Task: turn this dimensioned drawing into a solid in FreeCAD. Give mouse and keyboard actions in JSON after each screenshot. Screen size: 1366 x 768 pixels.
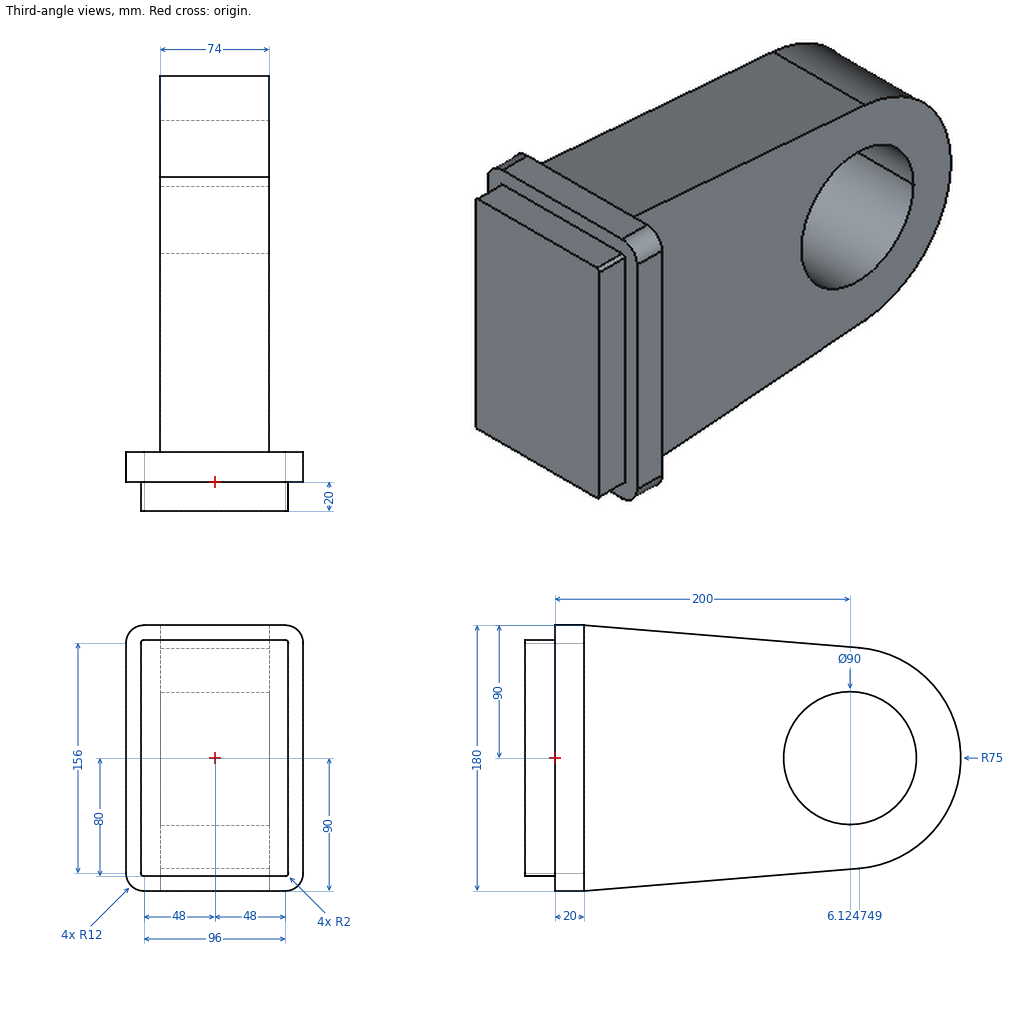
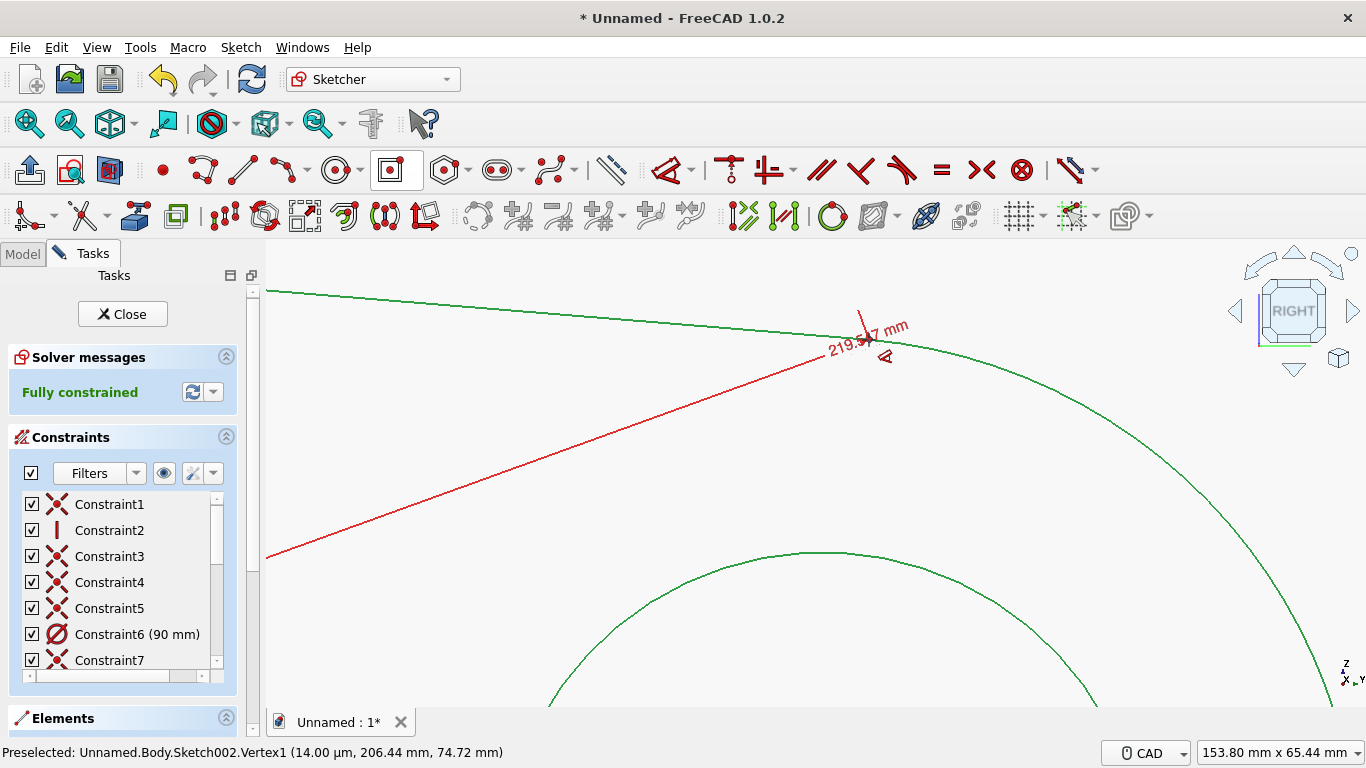
{"action": "scroll", "coordinate": [869, 342], "scroll_direction": "down", "scroll_amount": 7}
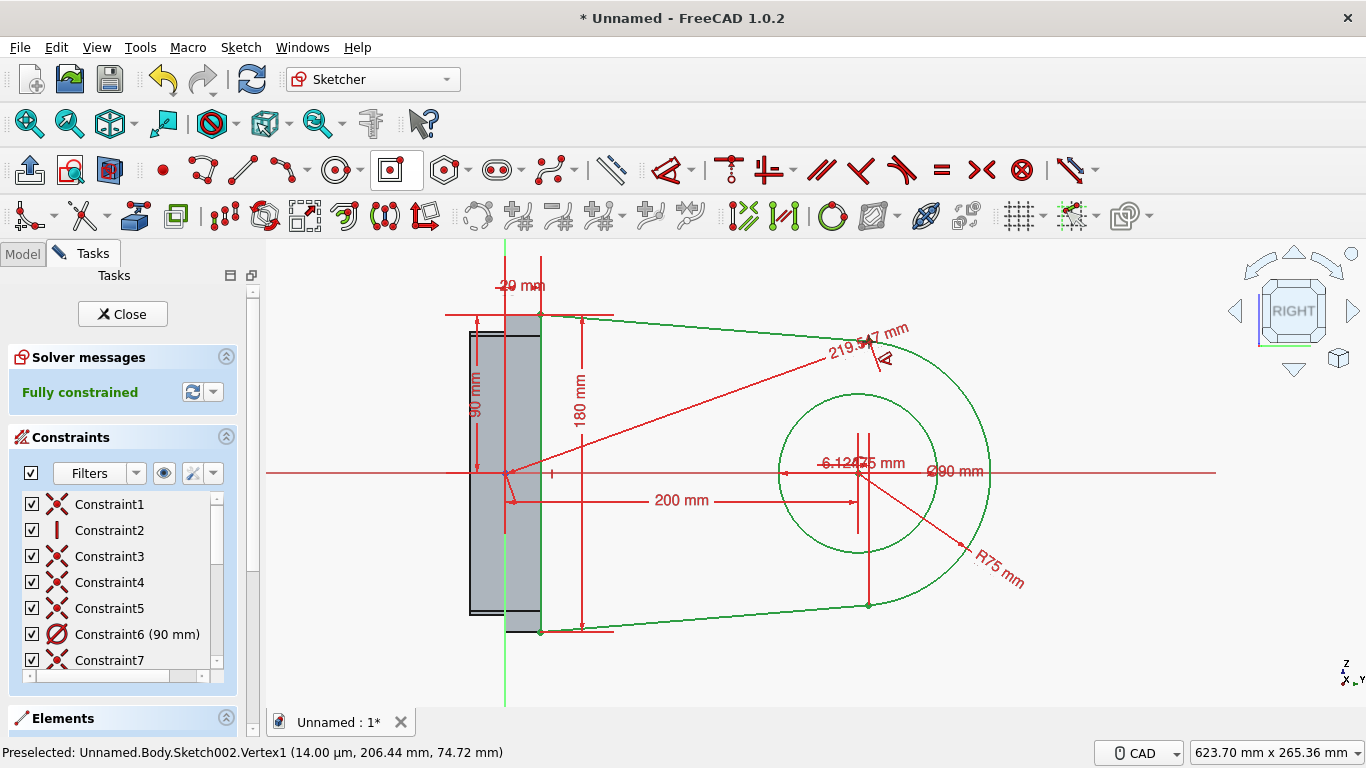
{"action": "scroll", "coordinate": [858, 473], "scroll_direction": "up", "scroll_amount": 7}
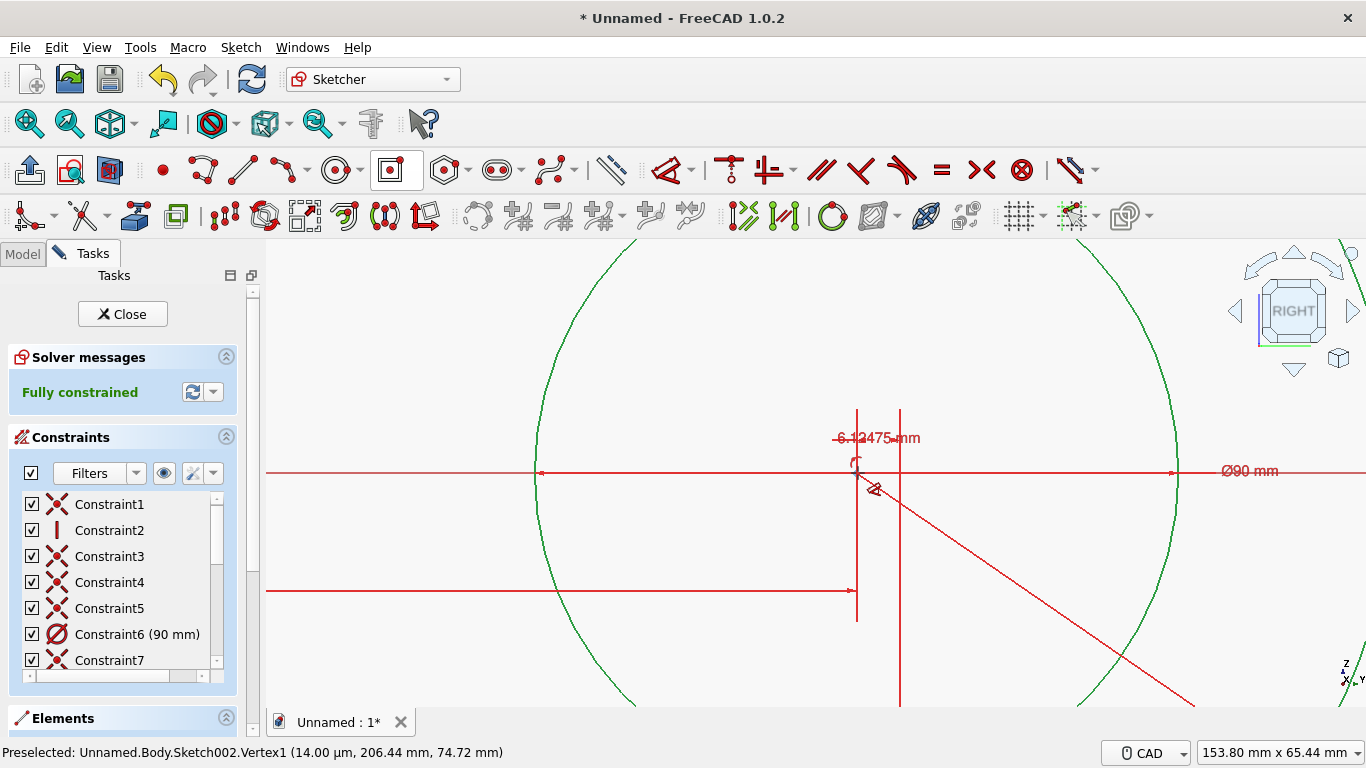
{"action": "left_click", "coordinate": [857, 473]}
{"action": "left_click", "coordinate": [880, 507]}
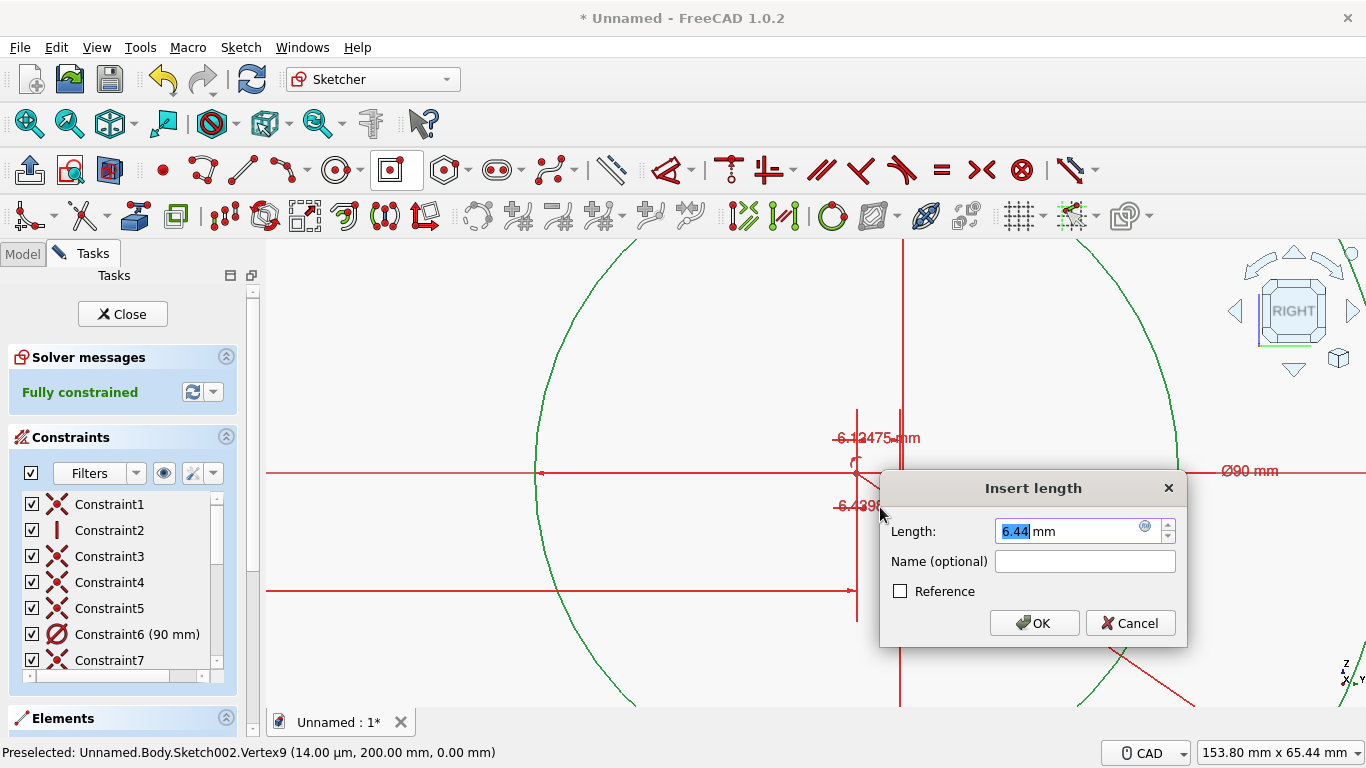
{"action": "type", "text": "6.124749"}
{"action": "key", "text": "Return"}
{"action": "key", "text": "Escape"}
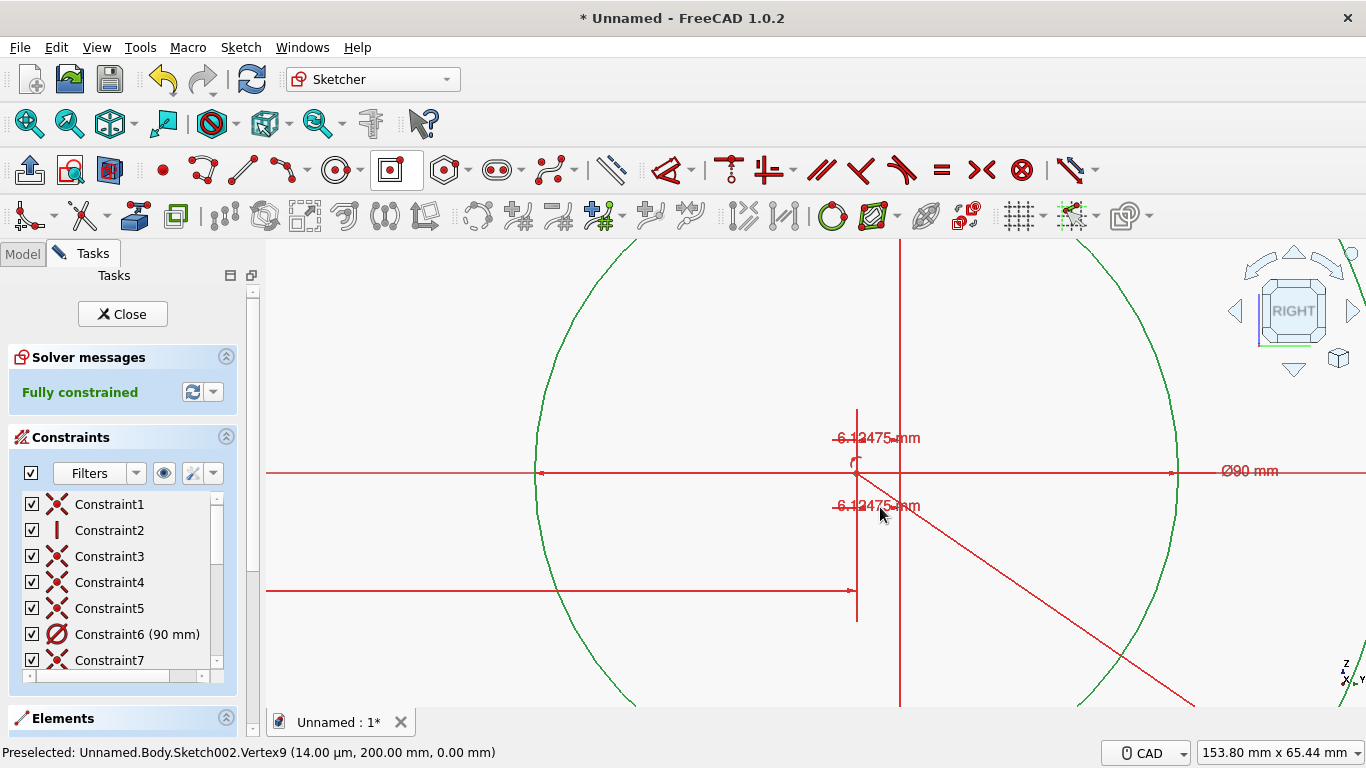
{"action": "left_click", "coordinate": [123, 314]}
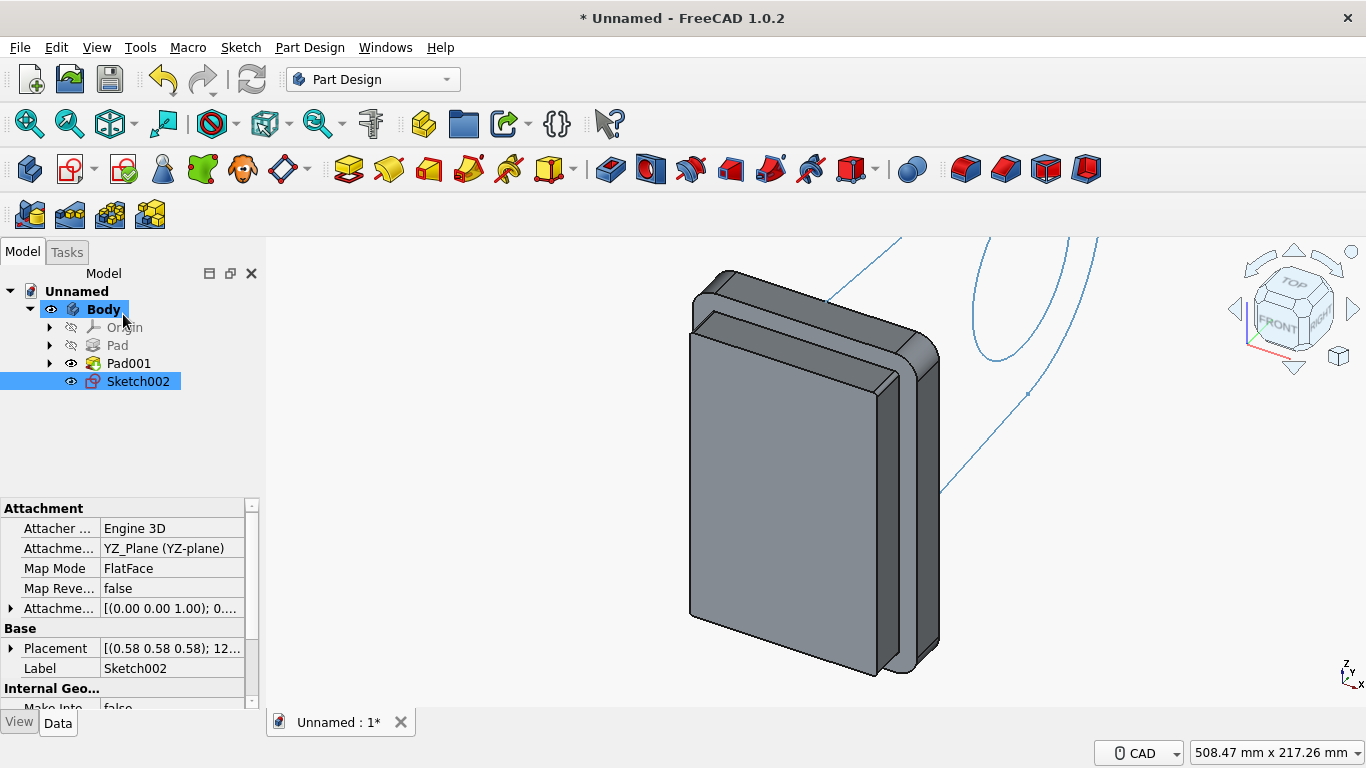
{"action": "left_click", "coordinate": [350, 170]}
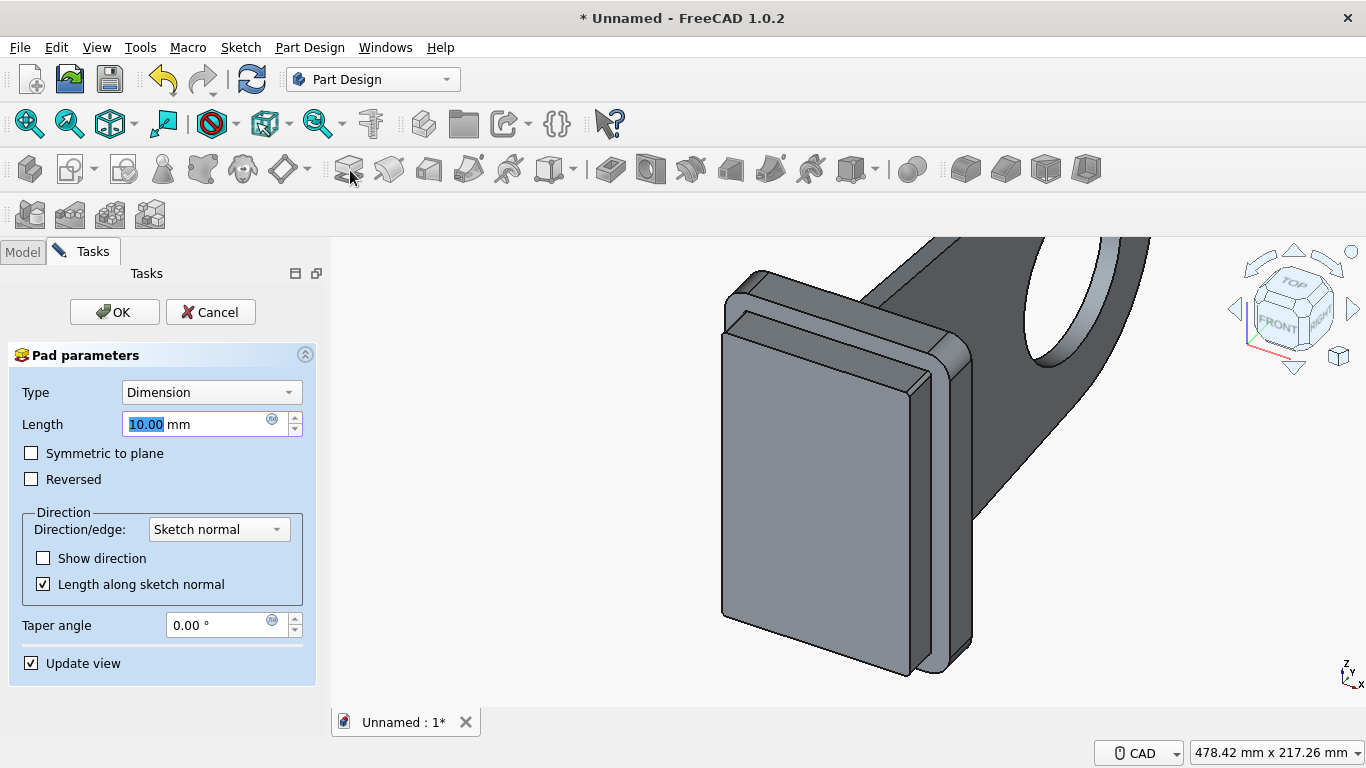
{"action": "type", "text": "74"}
{"action": "key", "text": "Tab"}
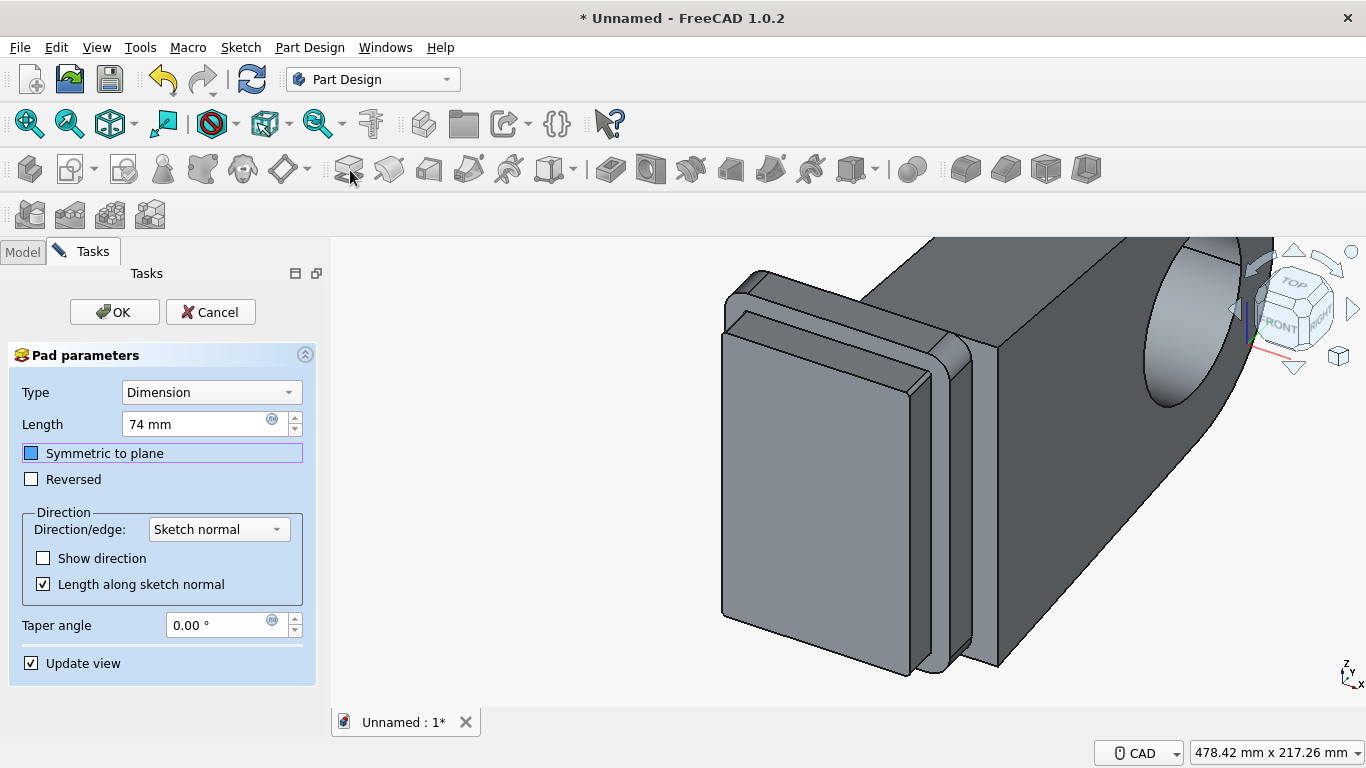
{"action": "left_click", "coordinate": [30, 453]}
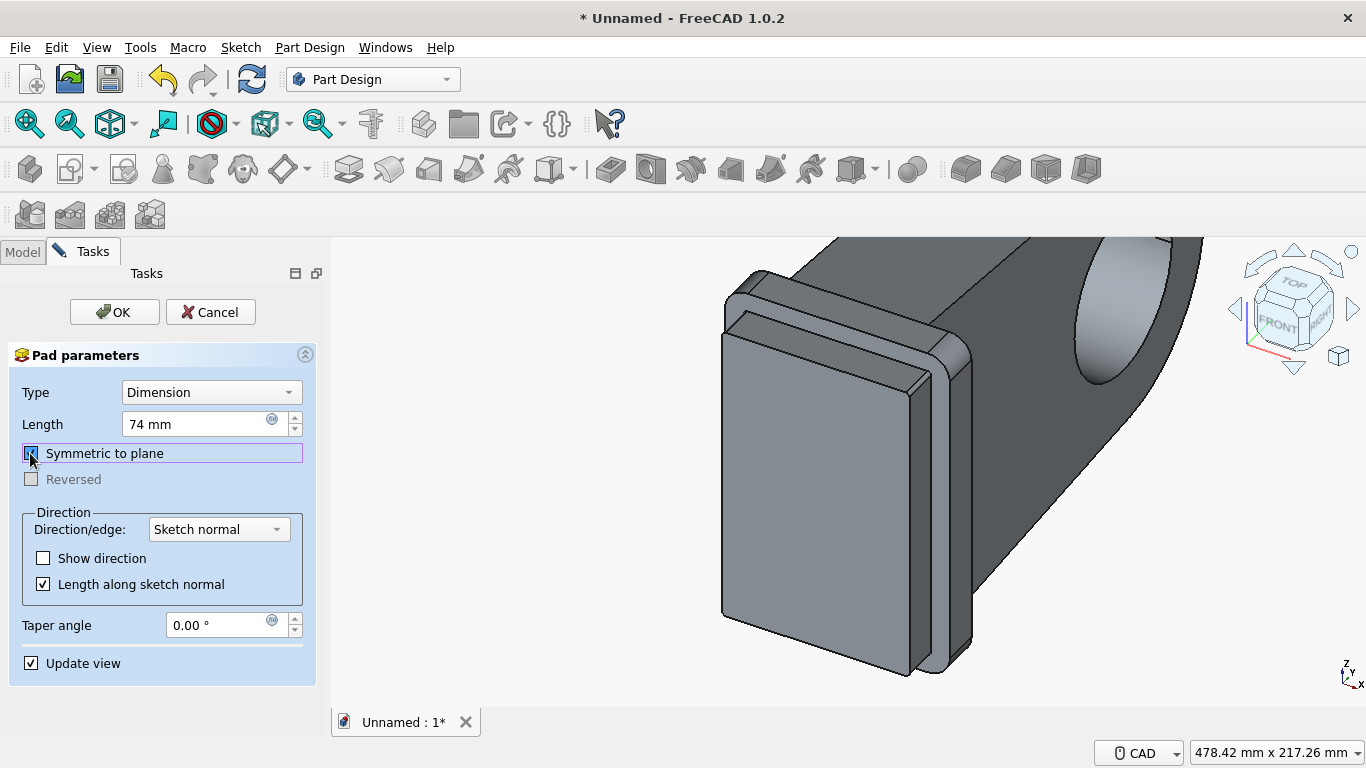
{"action": "left_click", "coordinate": [115, 312]}